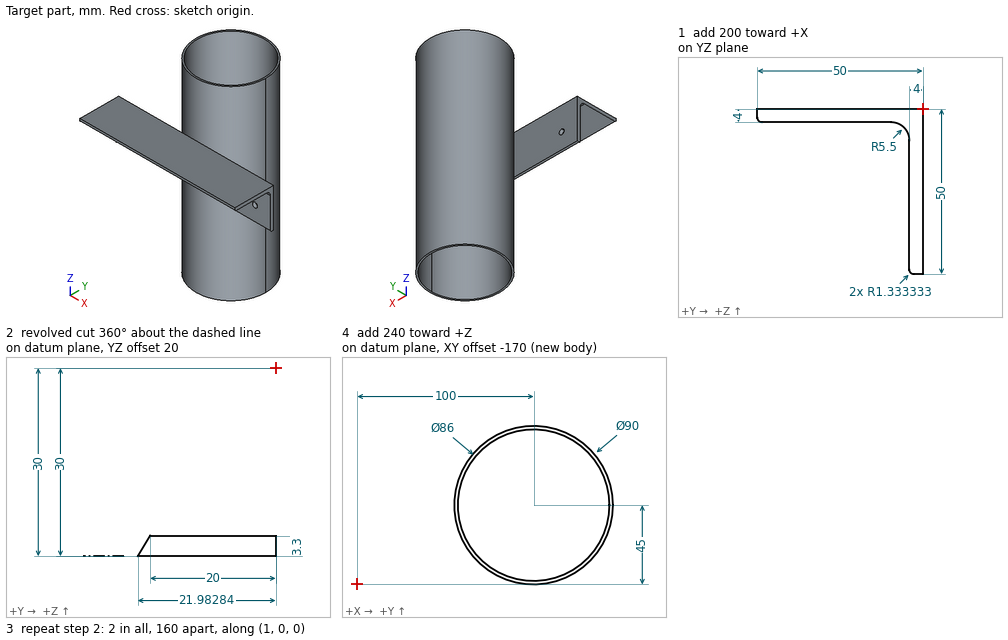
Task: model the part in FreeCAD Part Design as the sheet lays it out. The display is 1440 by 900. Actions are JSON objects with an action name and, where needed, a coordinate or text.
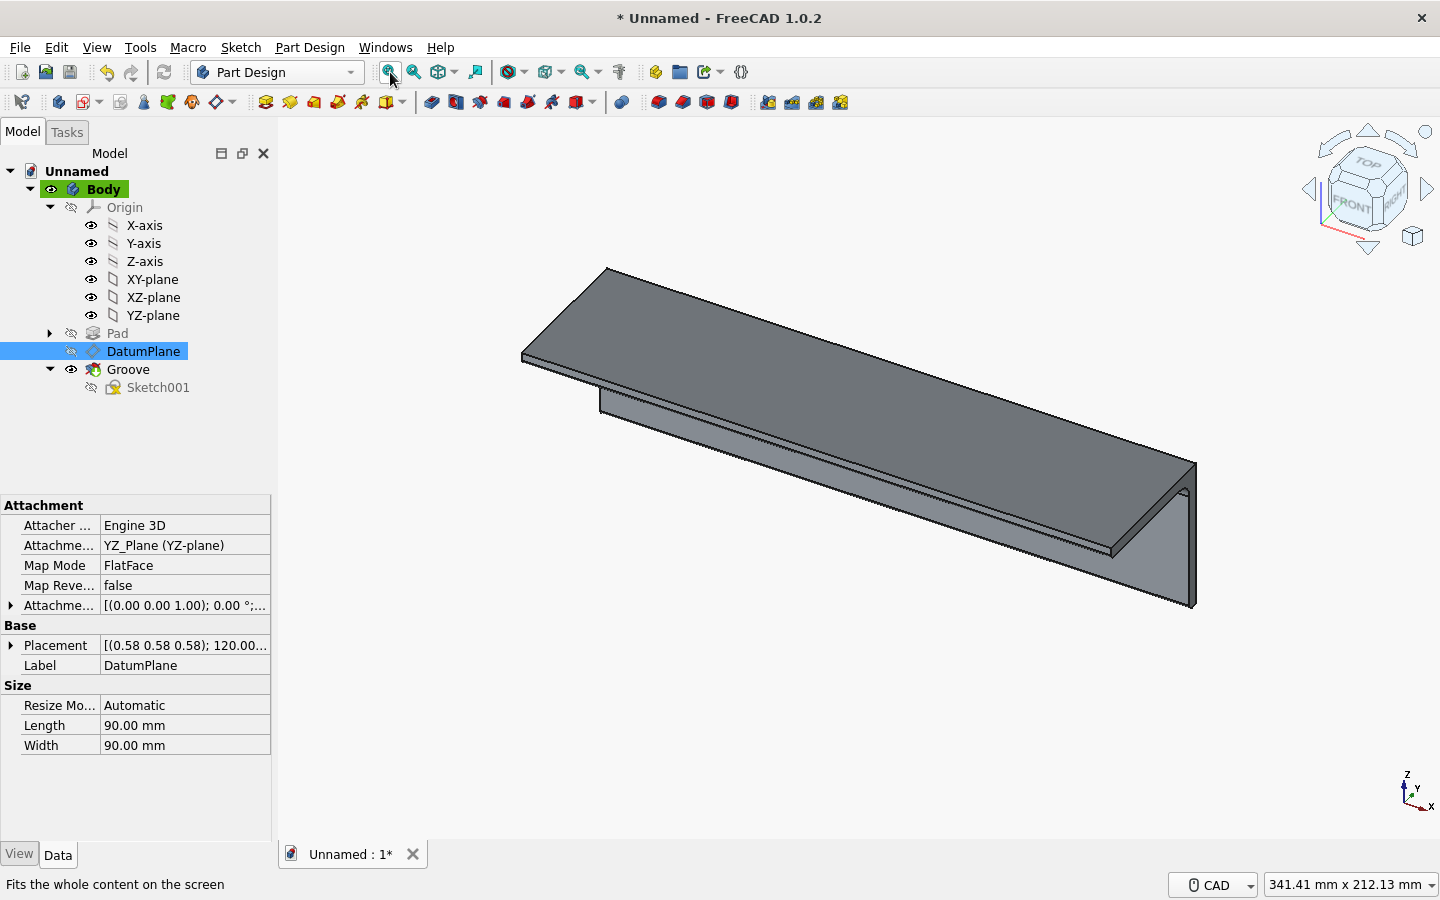
{"action": "left_click", "coordinate": [116, 369]}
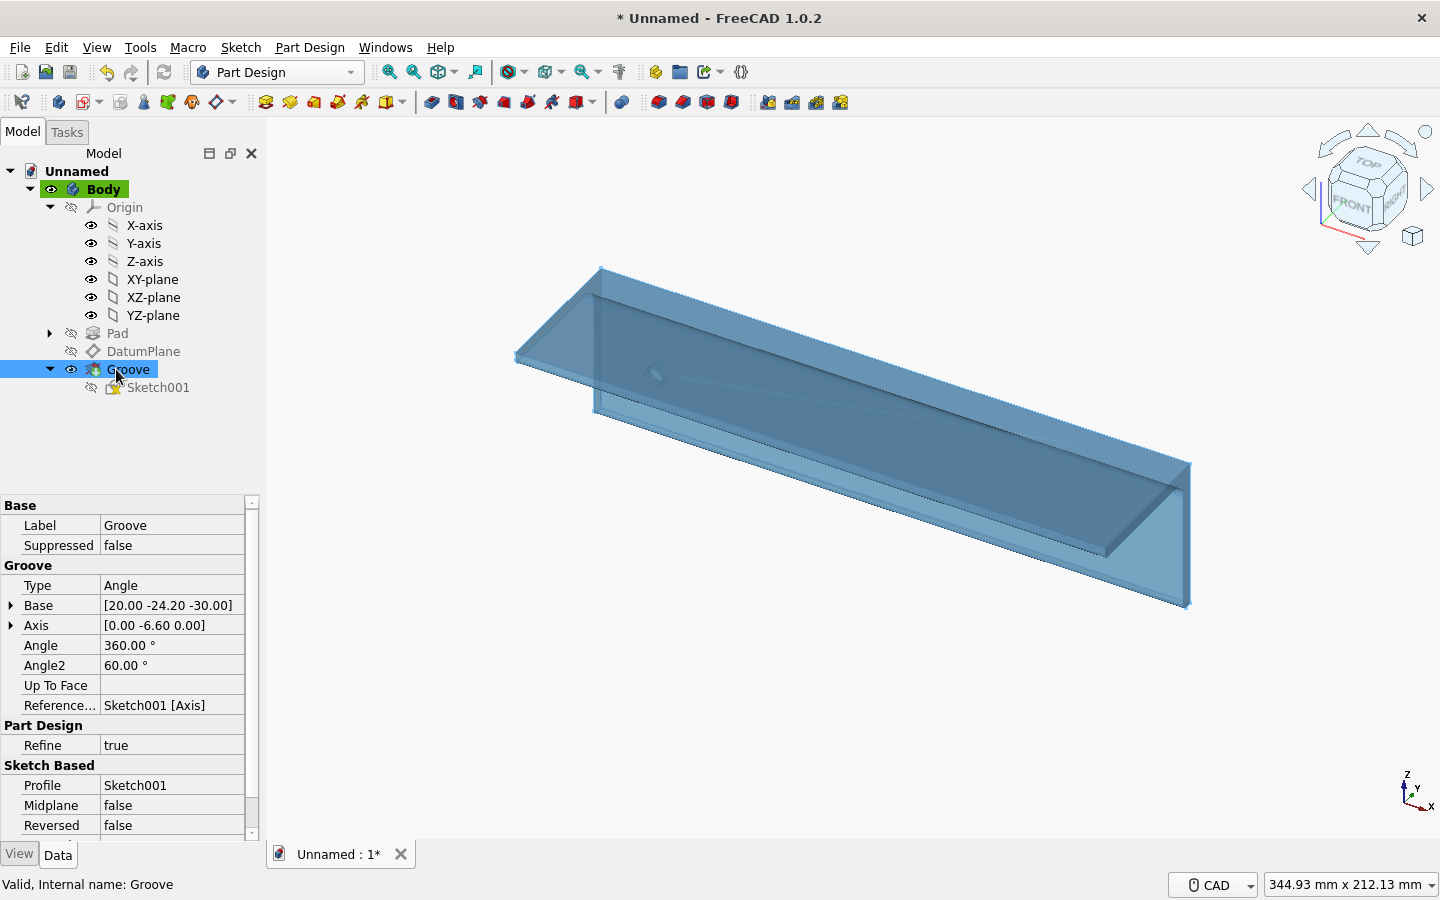
{"action": "left_click", "coordinate": [792, 102]}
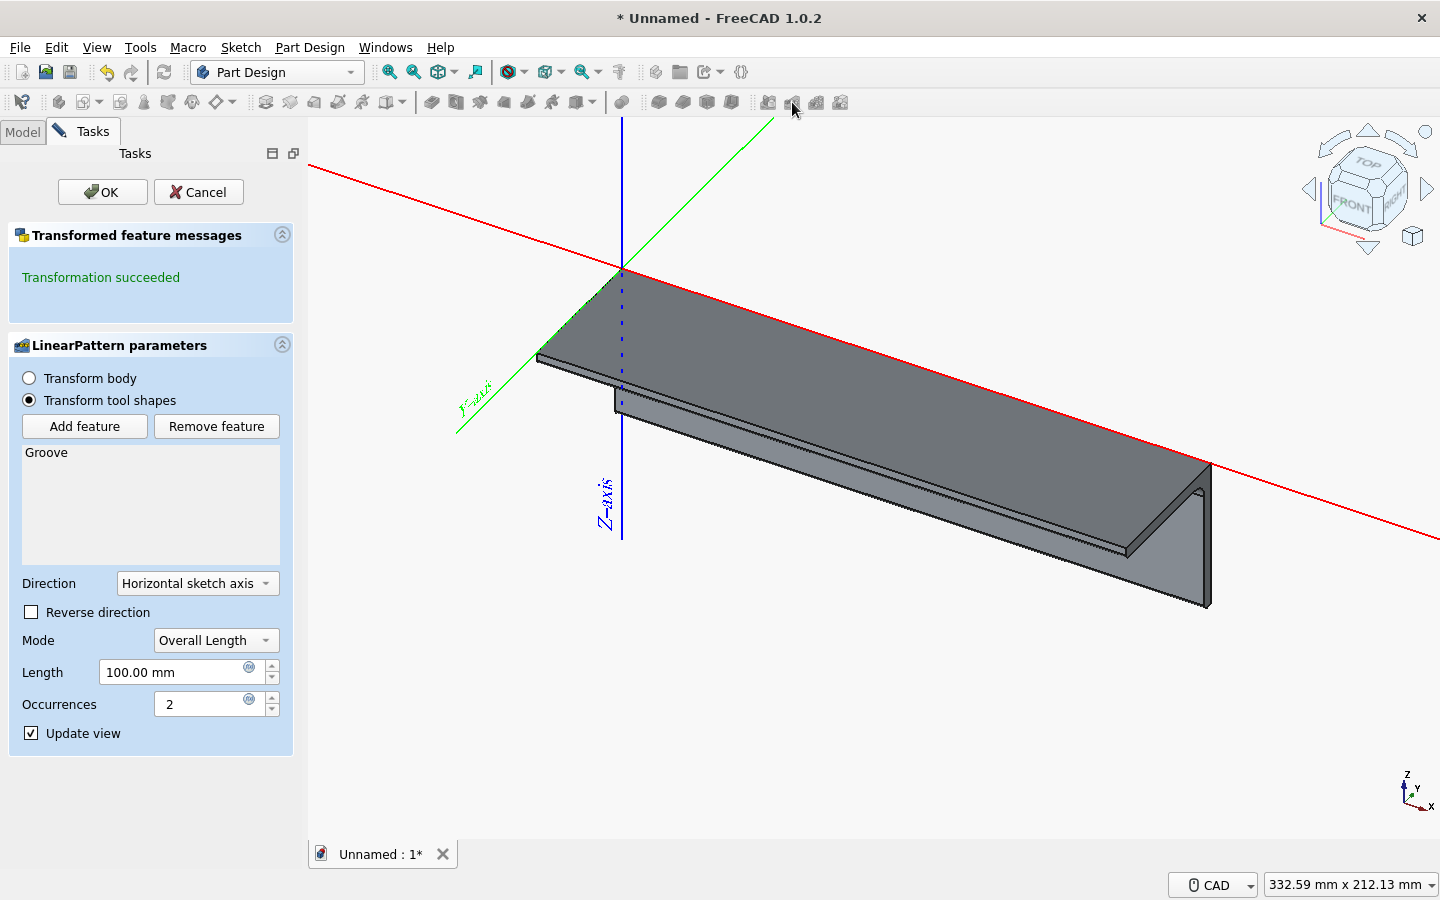
{"action": "left_click", "coordinate": [198, 584]}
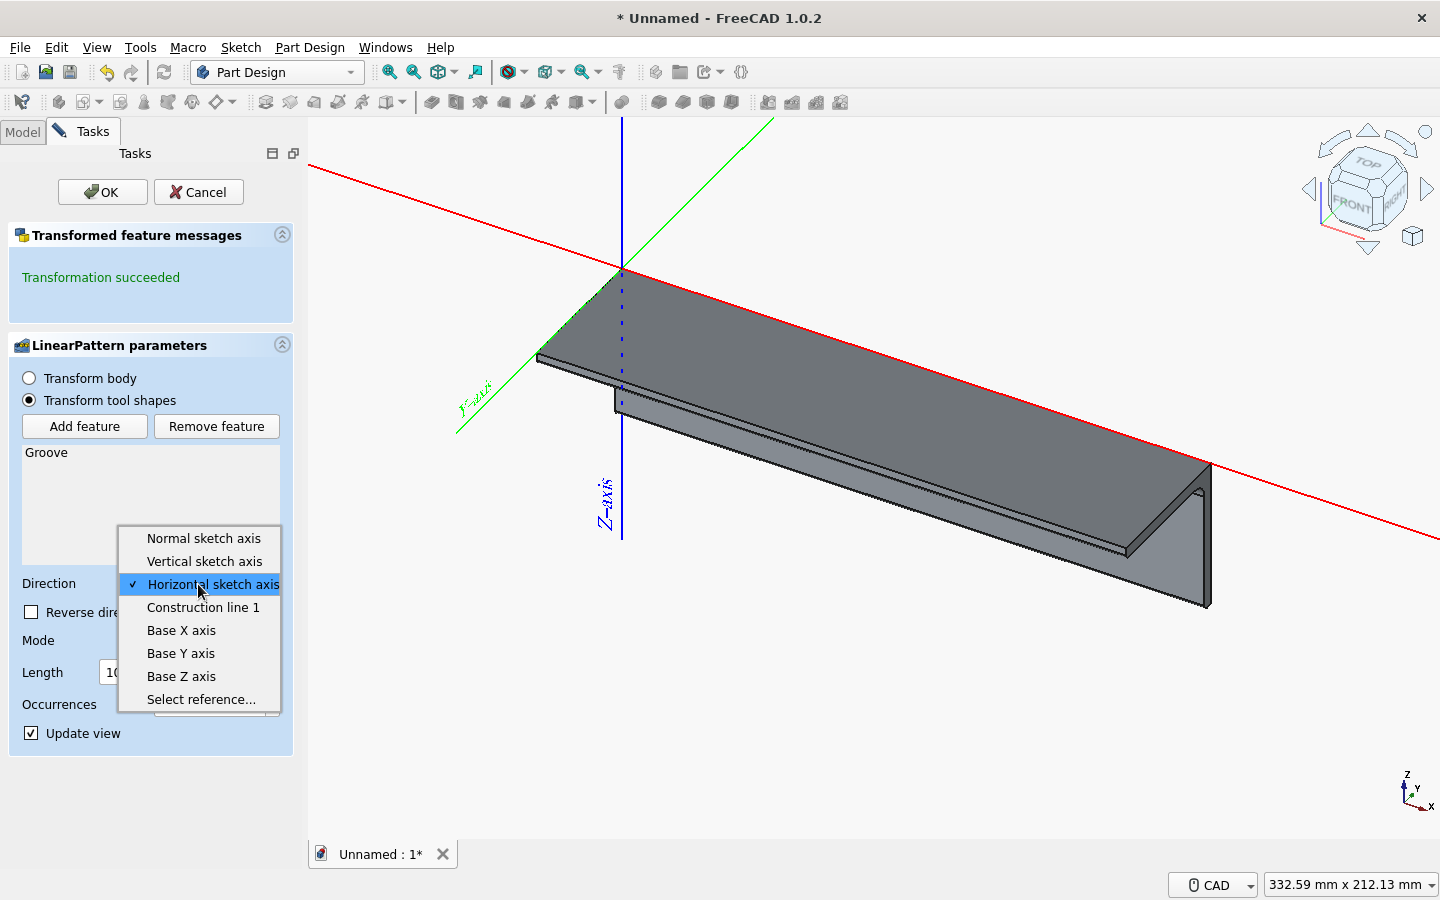
{"action": "left_click", "coordinate": [198, 630]}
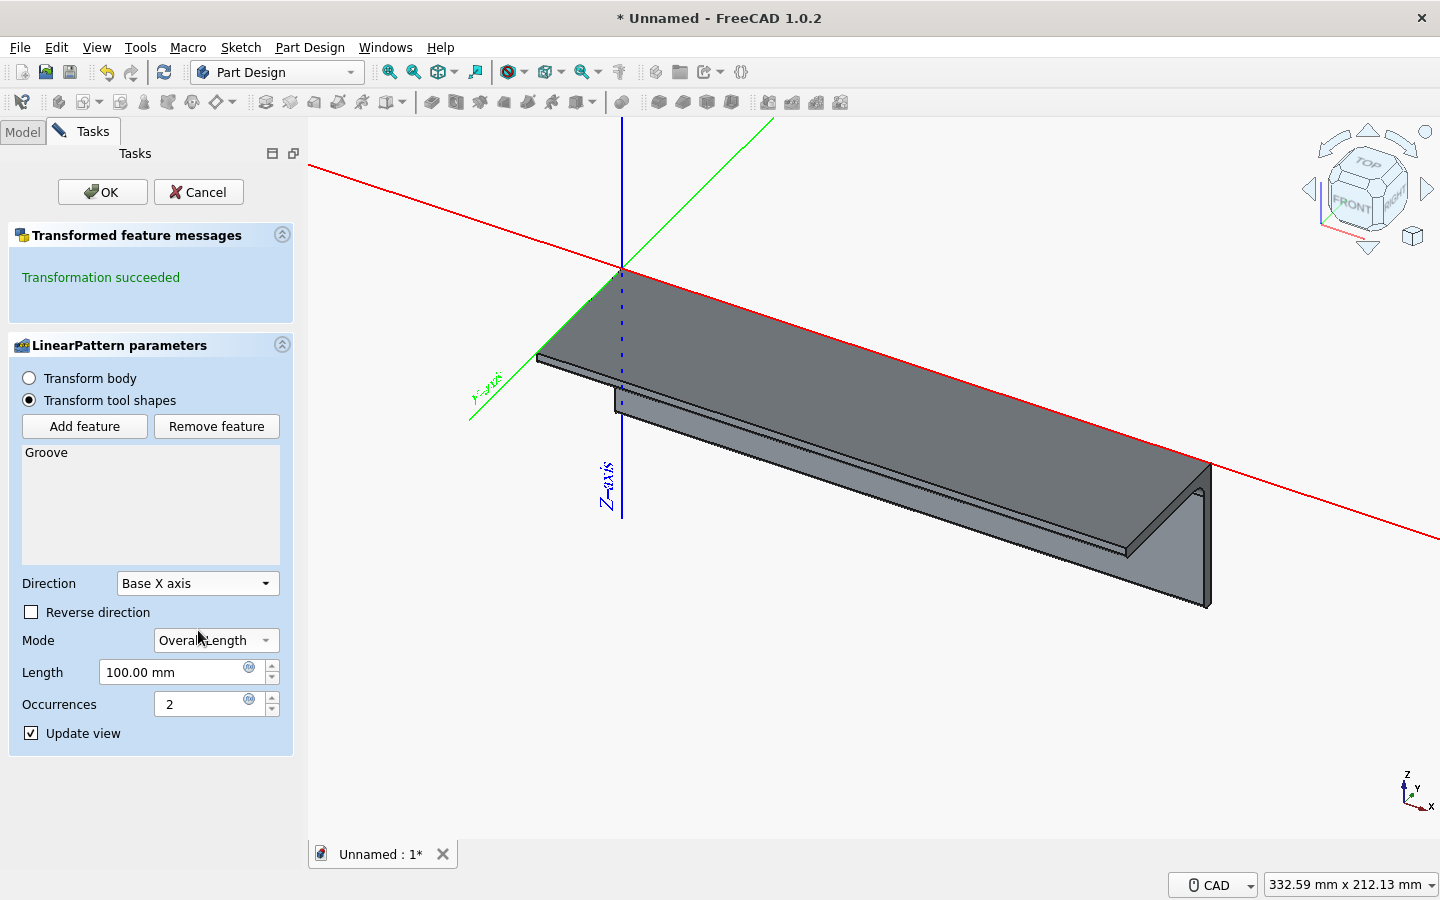
{"action": "left_click", "coordinate": [217, 640]}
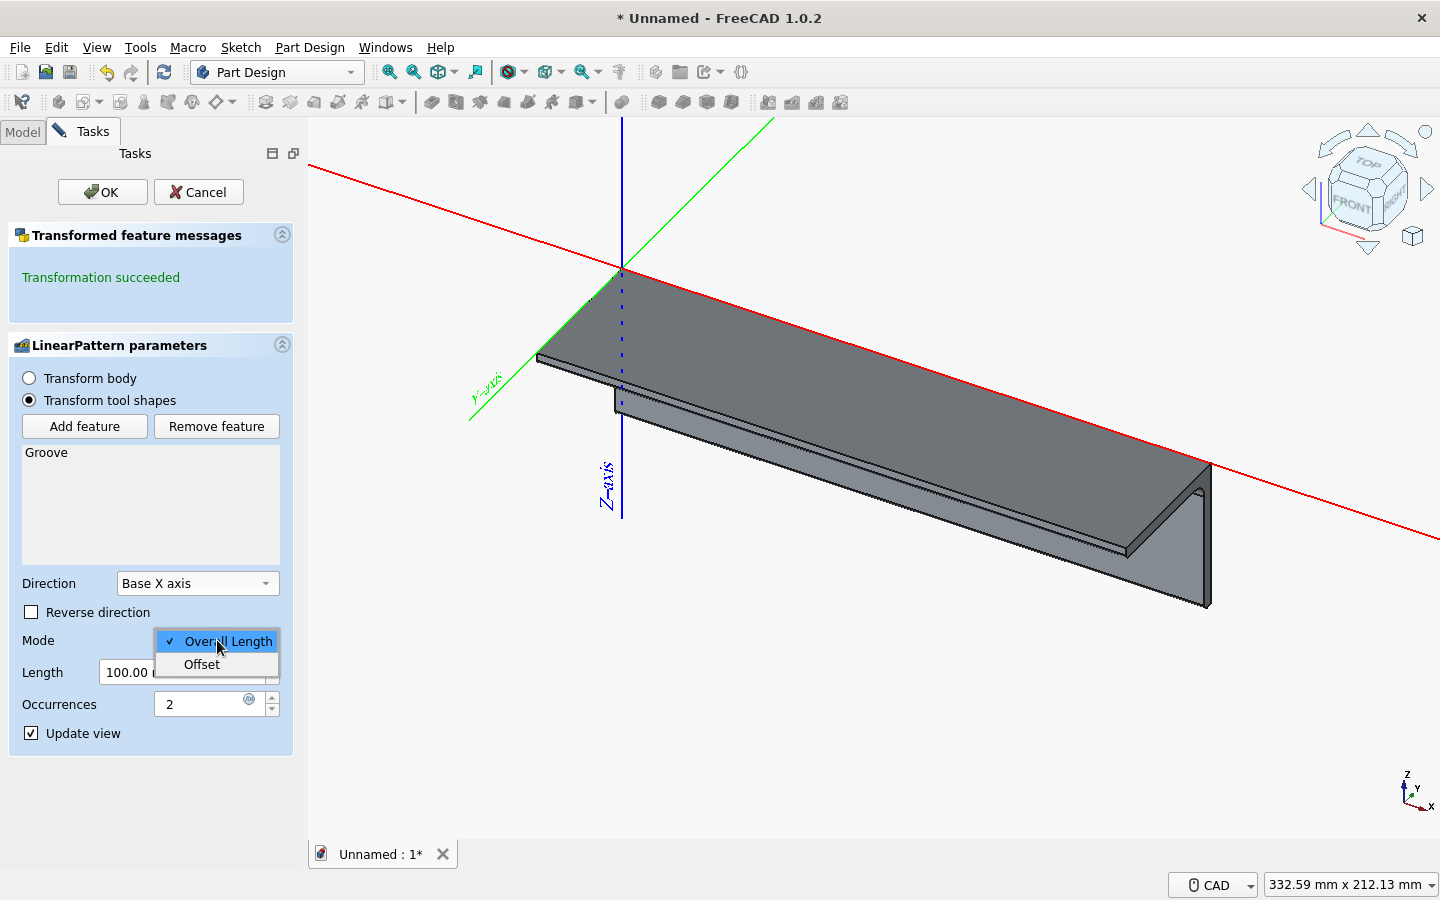
{"action": "left_click", "coordinate": [216, 664]}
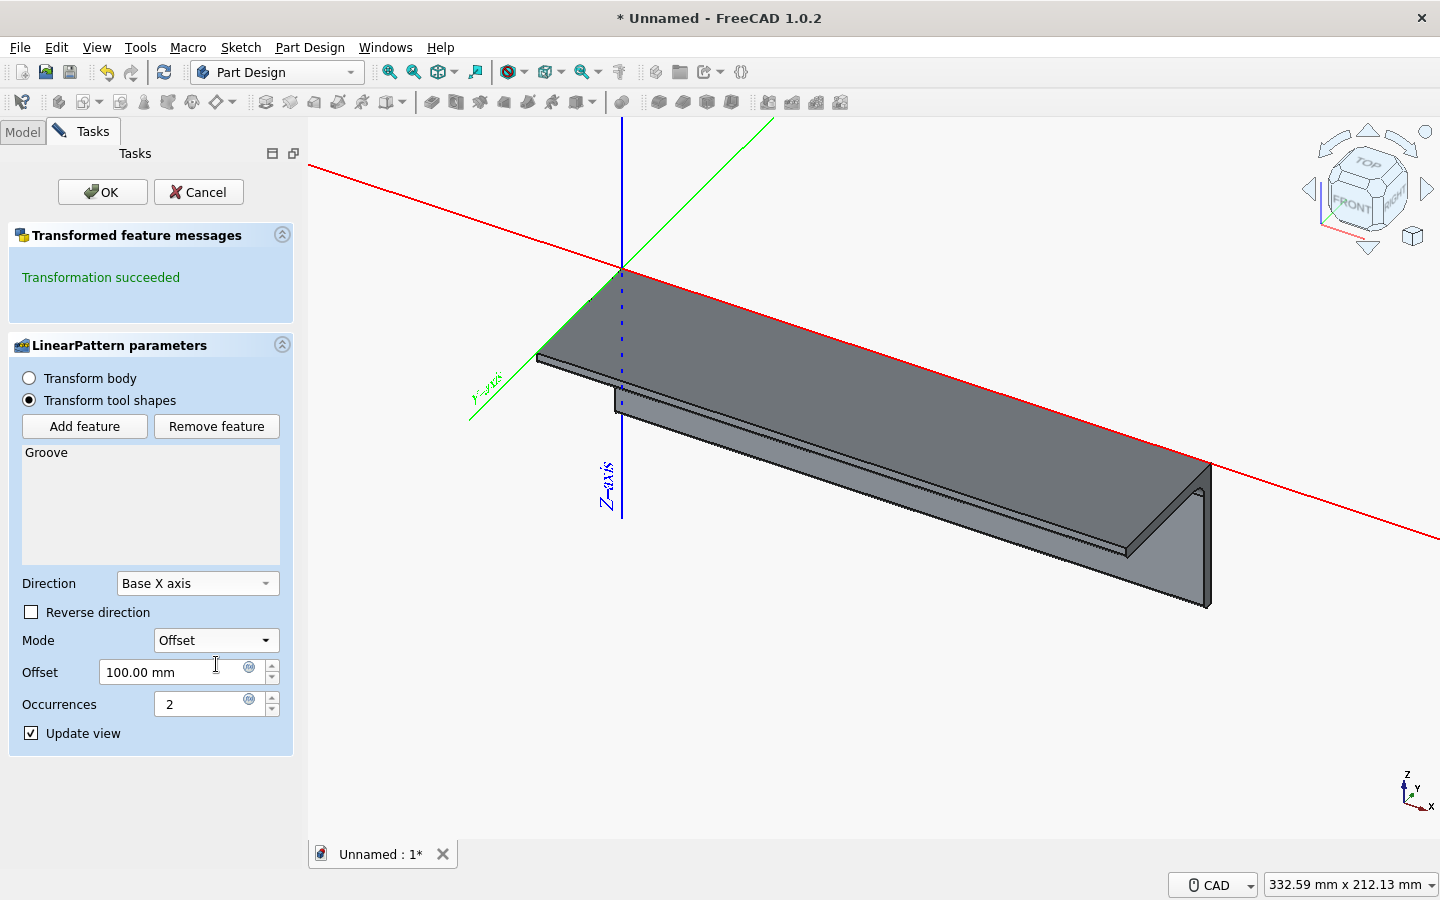
{"action": "triple_click", "coordinate": [182, 672]}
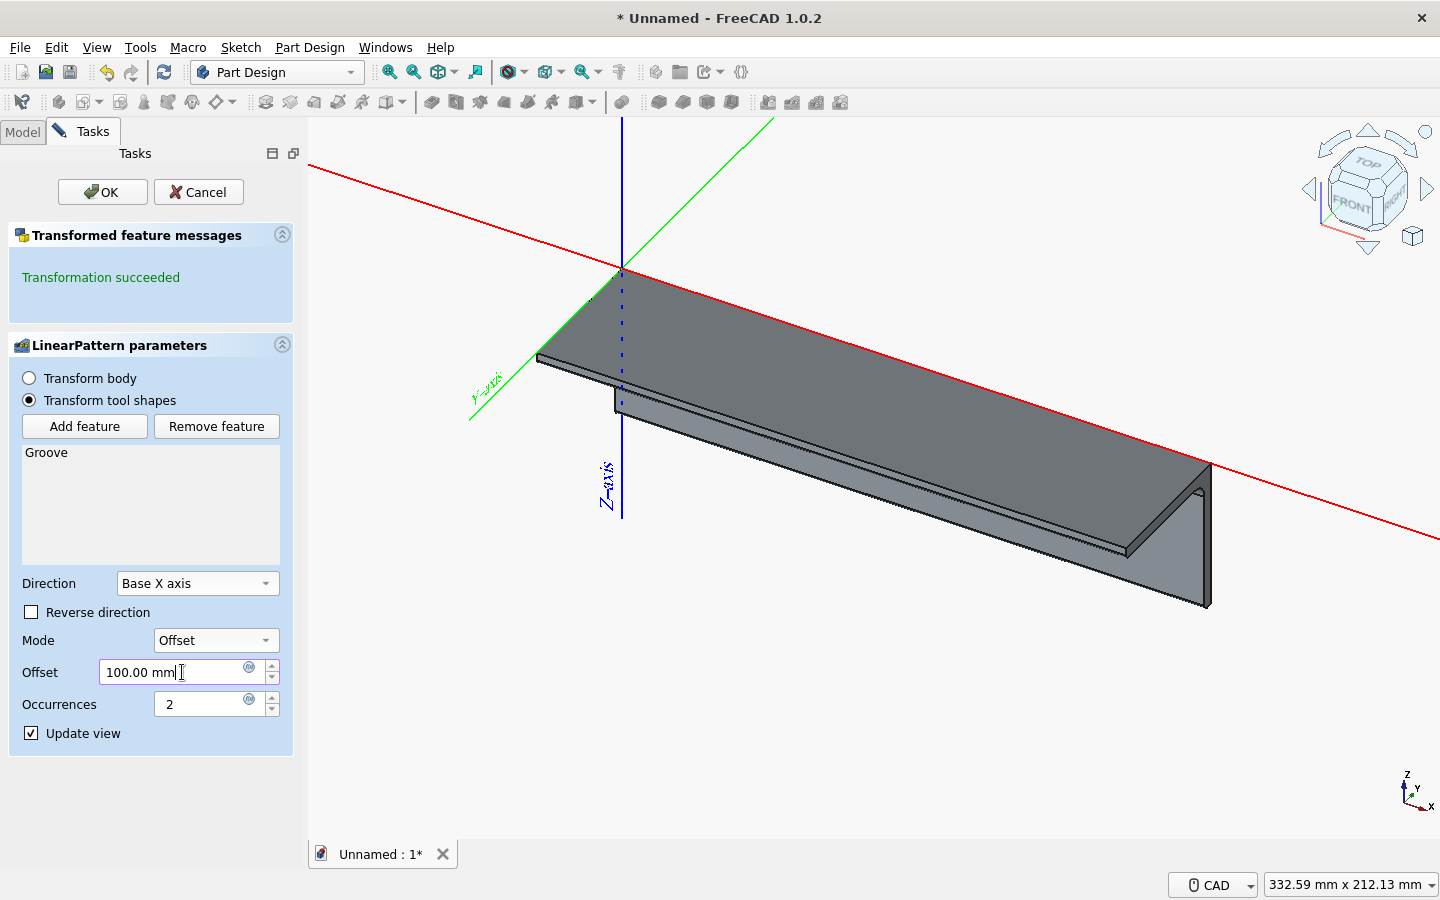
{"action": "type", "text": "160"}
{"action": "key", "text": "Tab"}